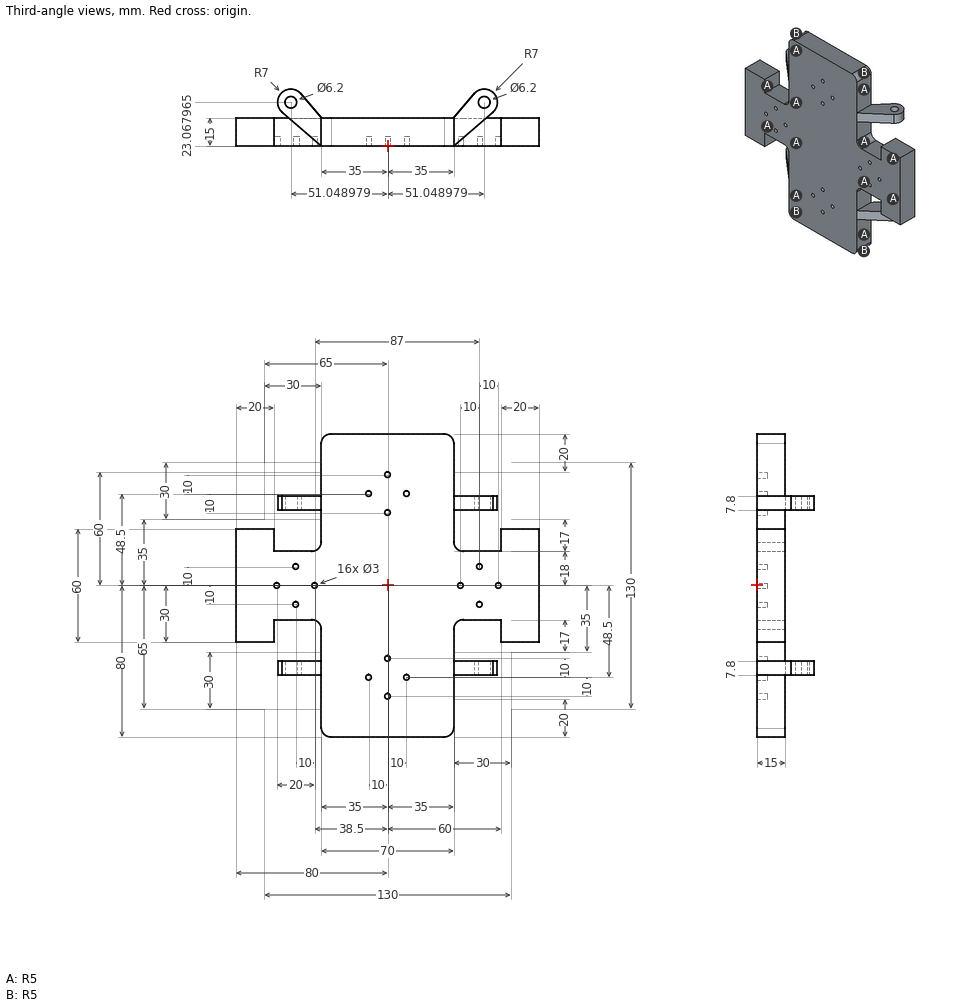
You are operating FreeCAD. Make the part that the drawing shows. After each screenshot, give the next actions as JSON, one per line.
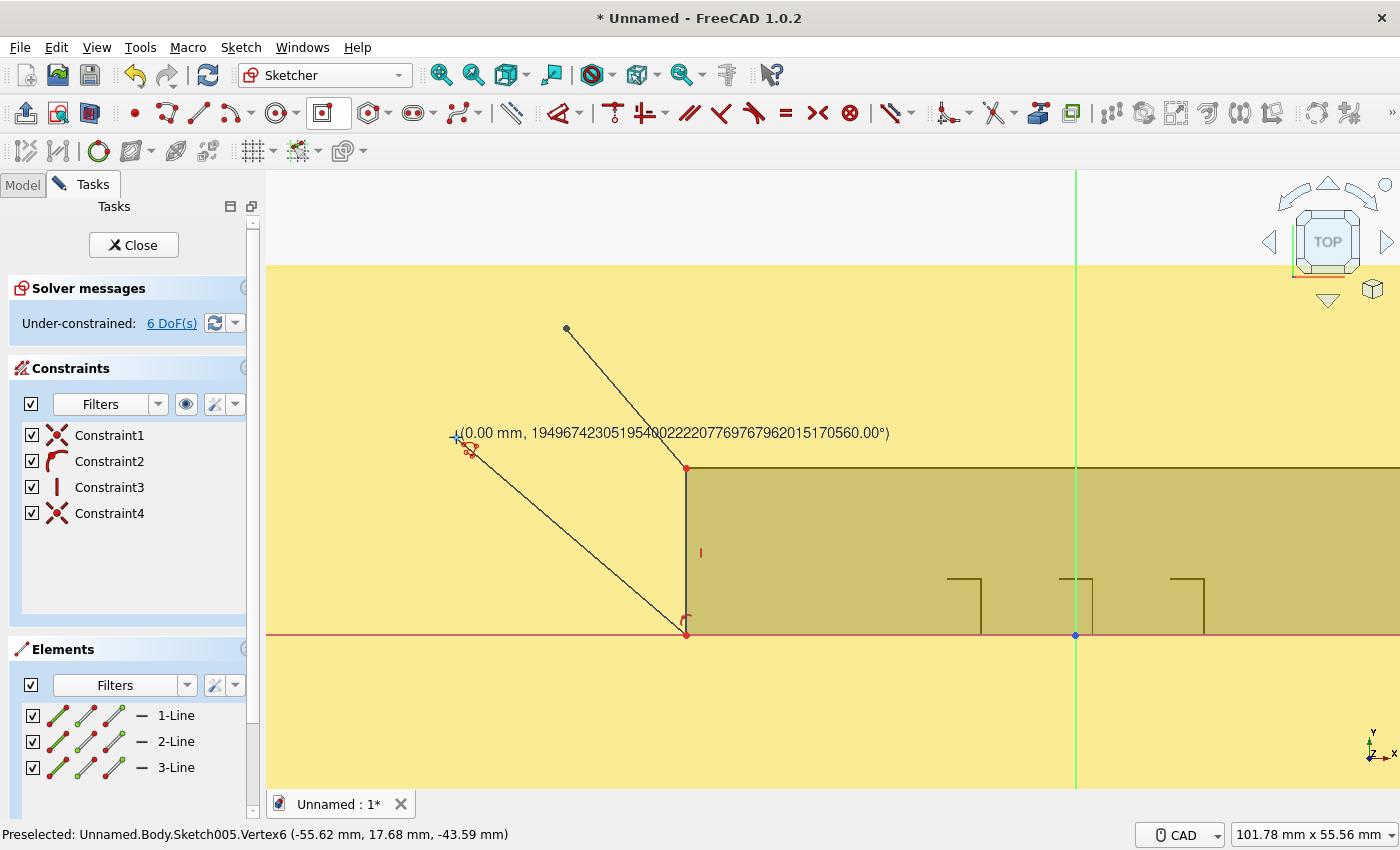
{"action": "key", "text": "g 3 a"}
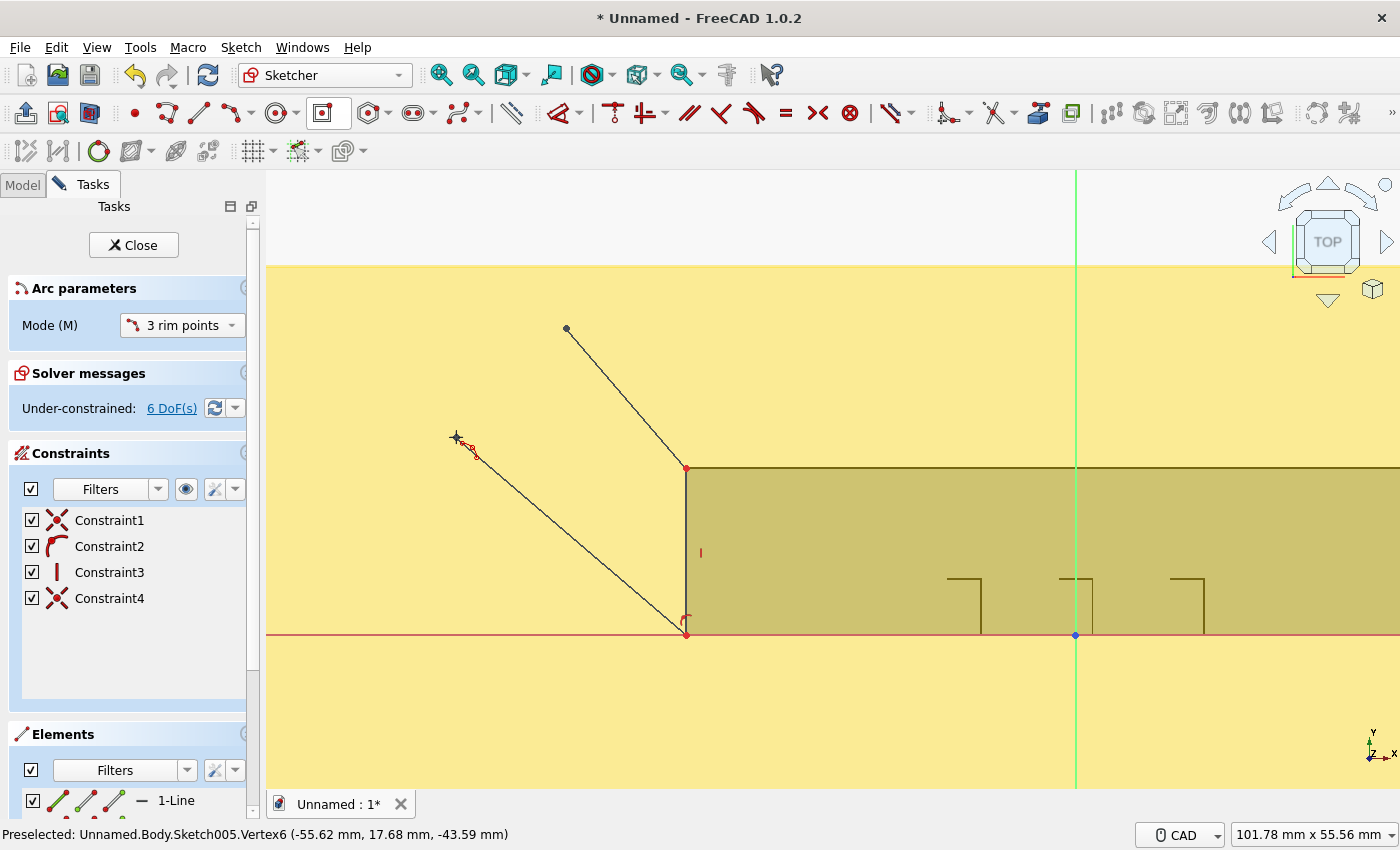
{"action": "left_click", "coordinate": [456, 438]}
{"action": "left_click", "coordinate": [566, 329]}
{"action": "left_click", "coordinate": [452, 323]}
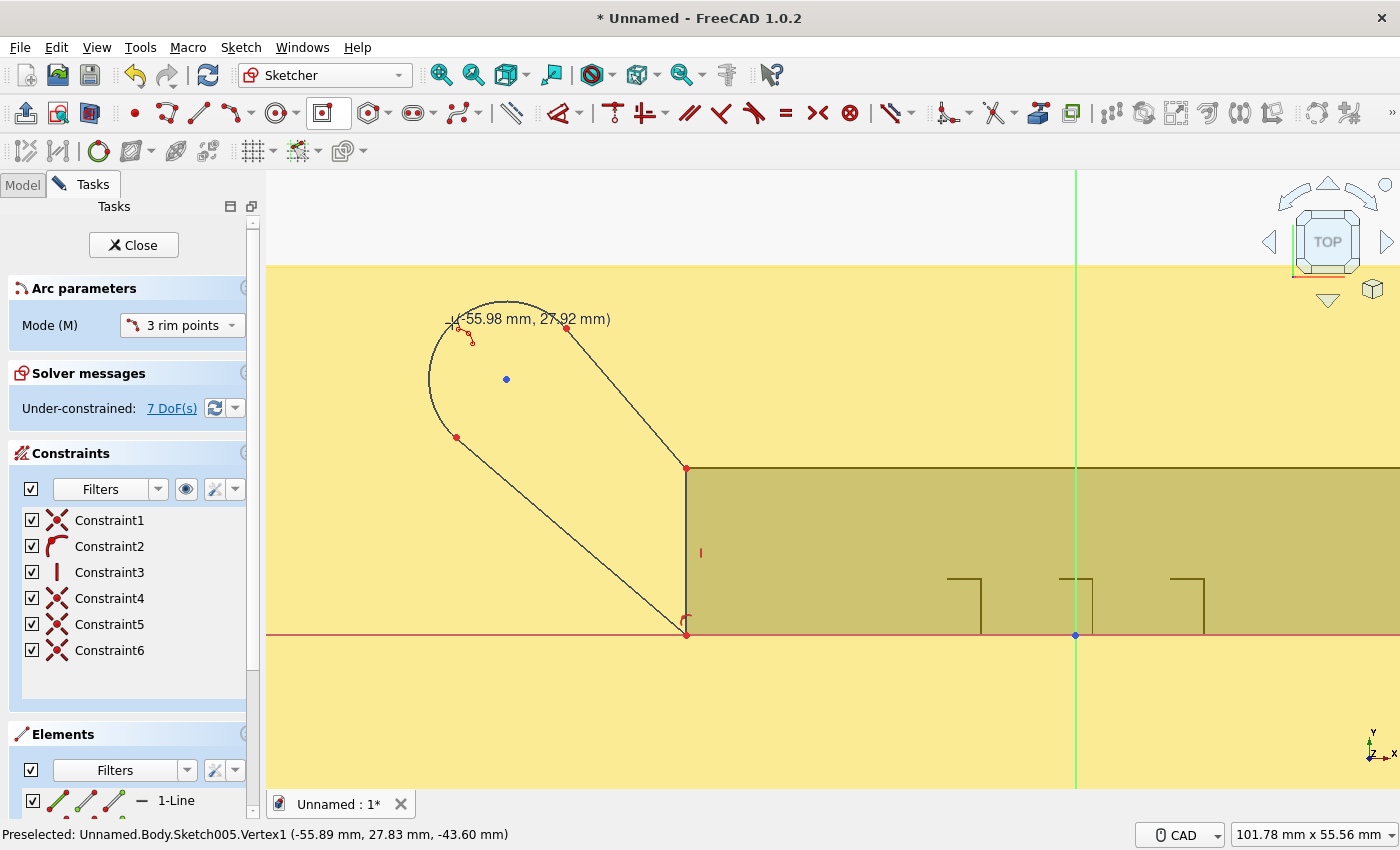
{"action": "key", "text": "g c"}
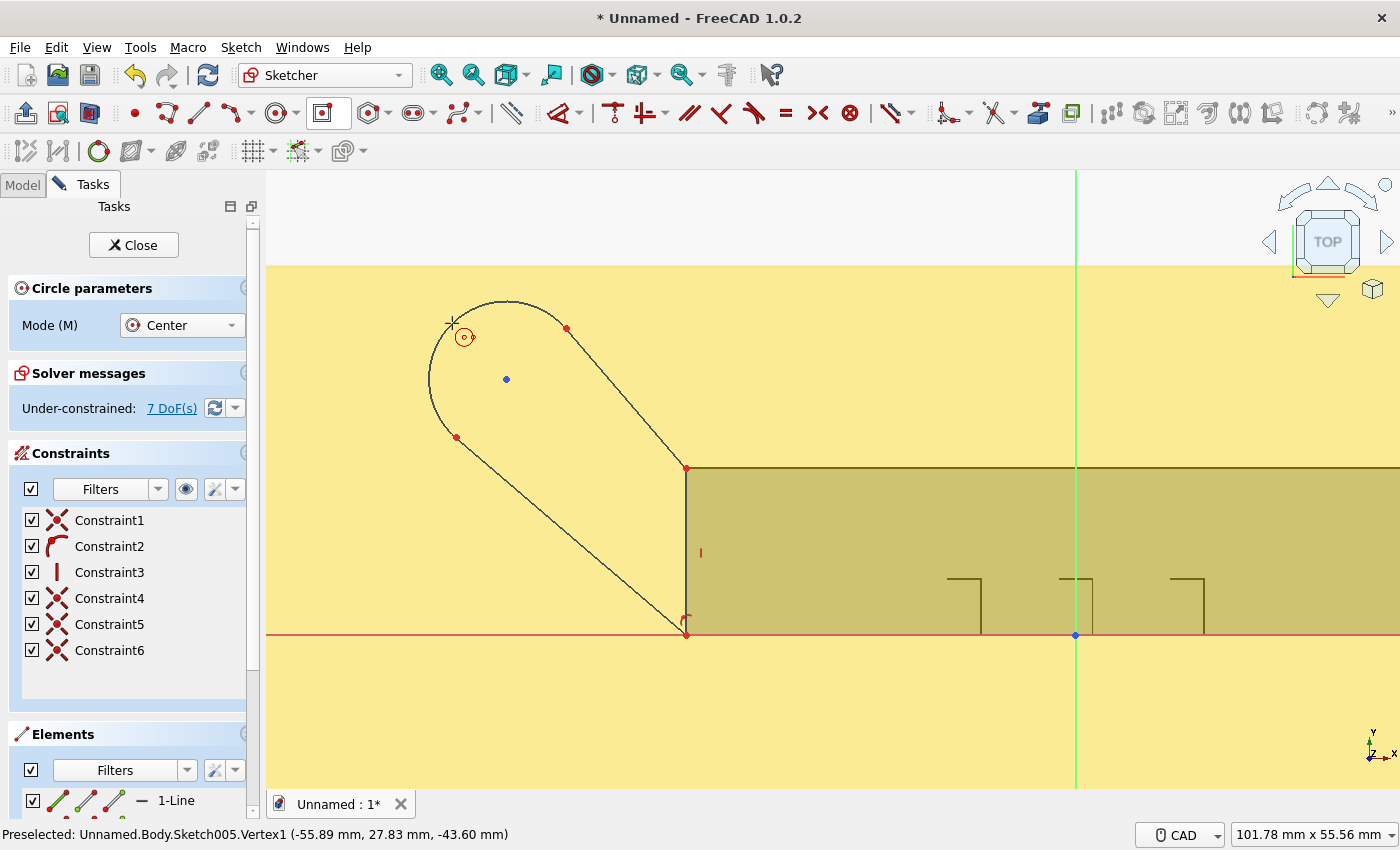
{"action": "left_click", "coordinate": [507, 378]}
{"action": "mouse_move", "coordinate": [531, 354]}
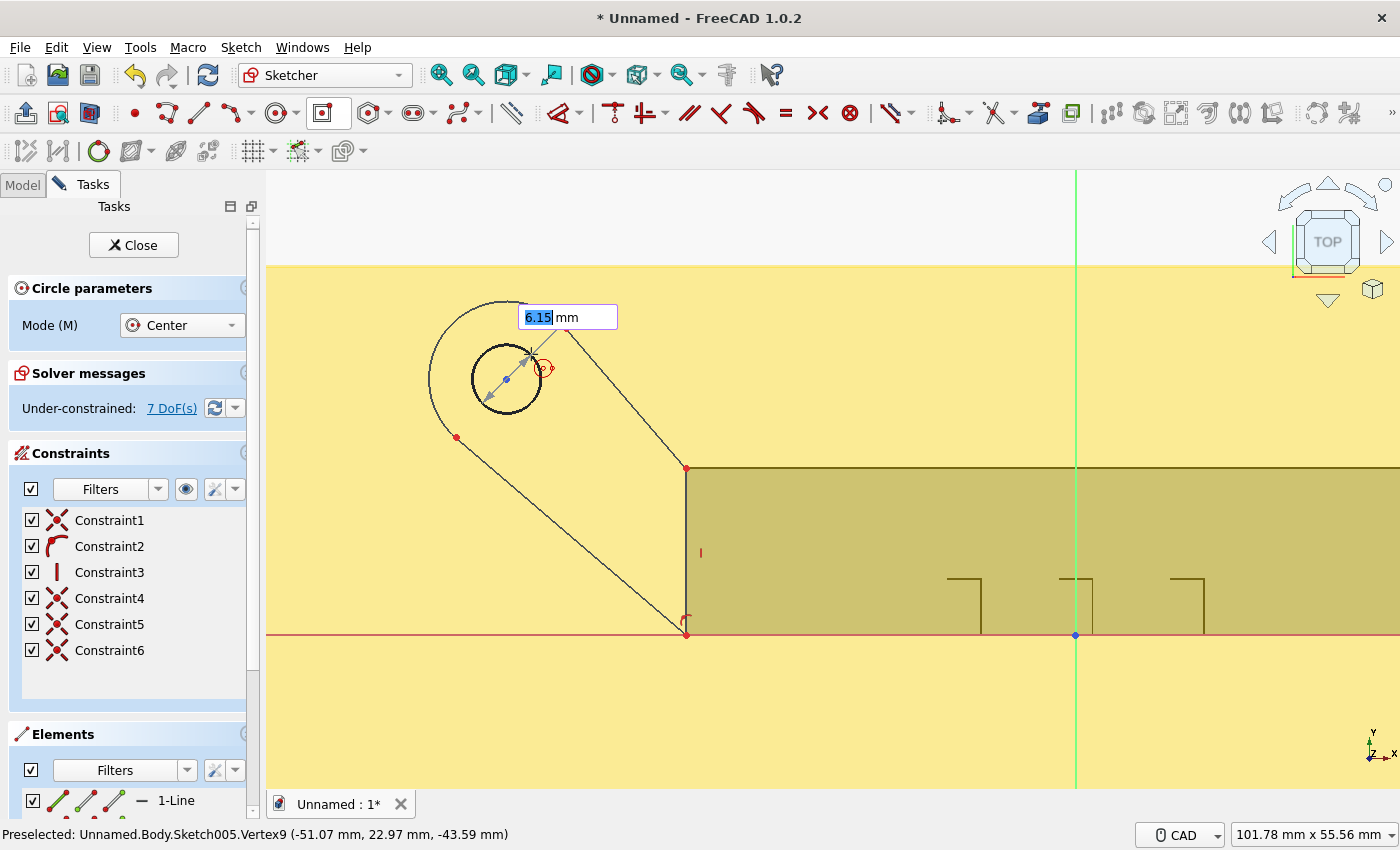
{"action": "type", "text": "6.2"}
{"action": "key", "text": "Return"}
{"action": "key", "text": "Escape"}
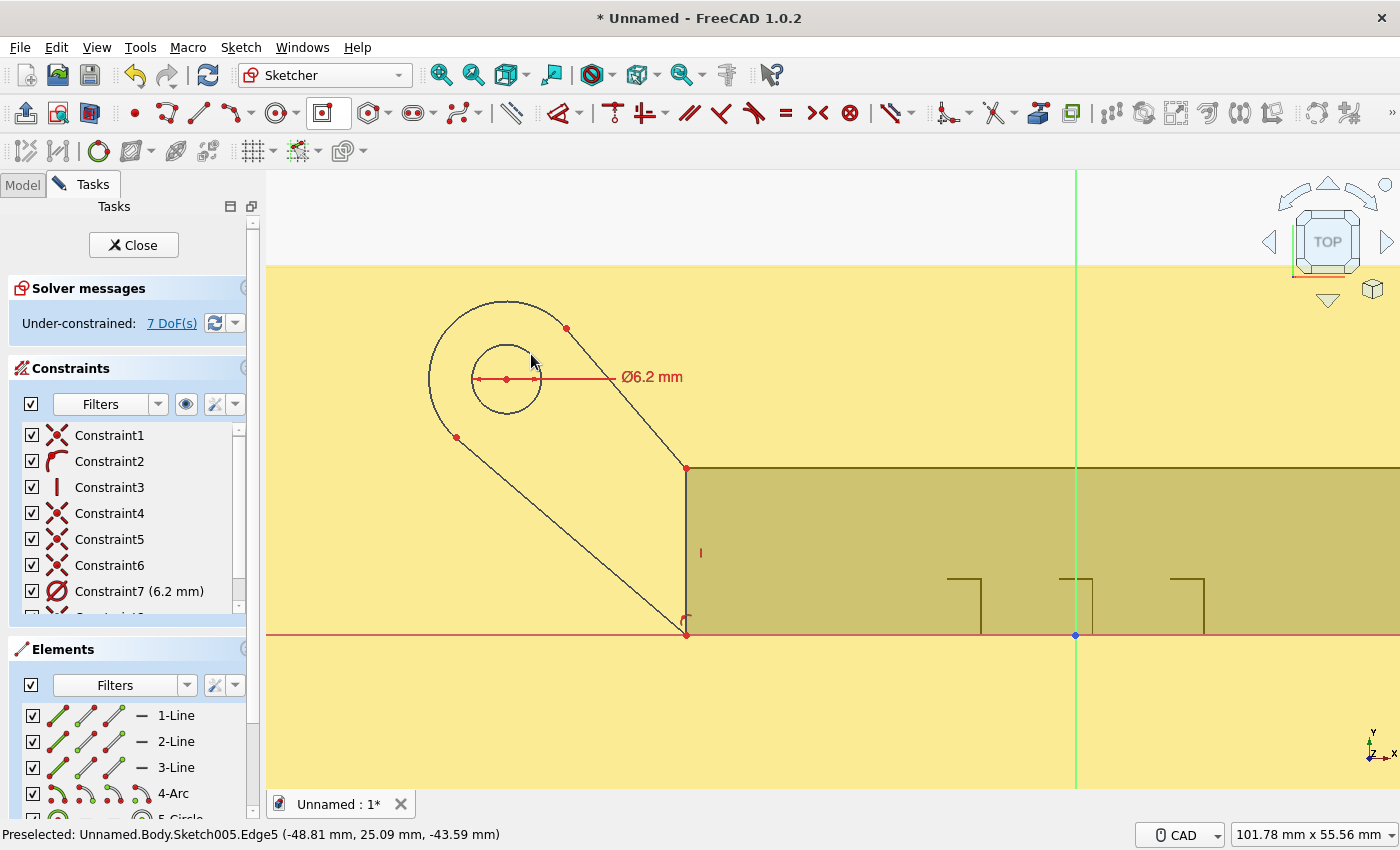
{"action": "left_click", "coordinate": [602, 371]}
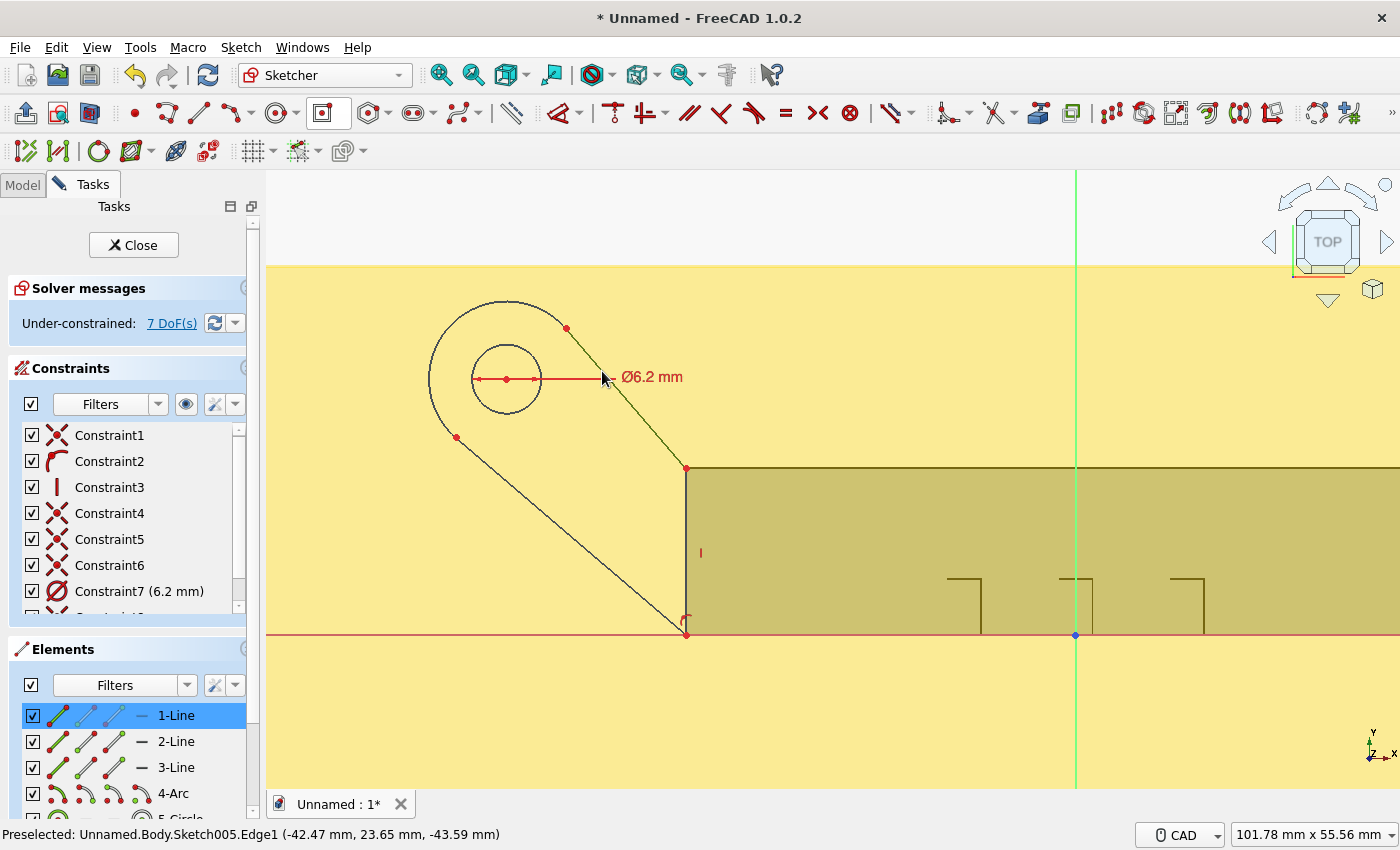
{"action": "left_click", "coordinate": [497, 302]}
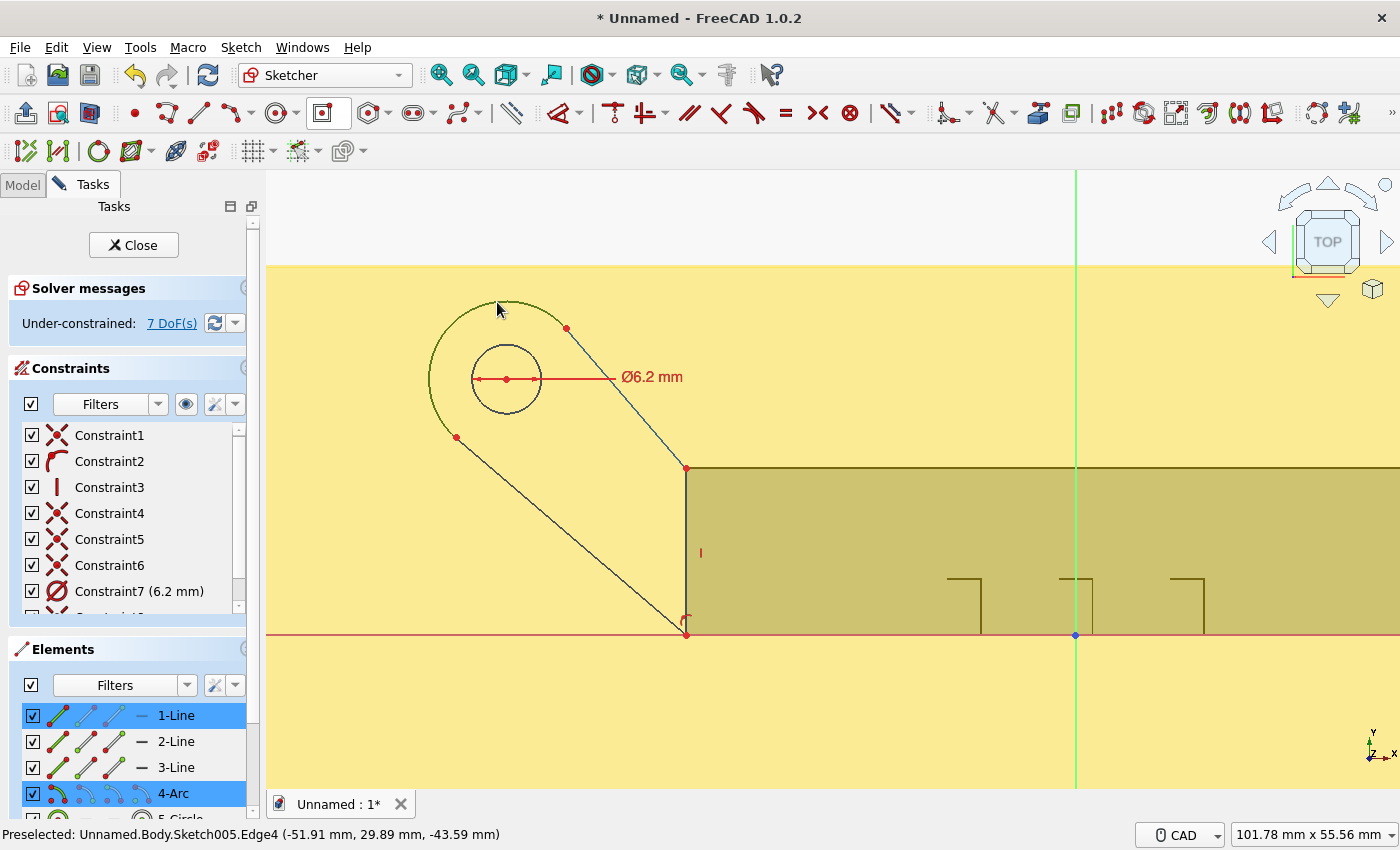
{"action": "key", "text": "t"}